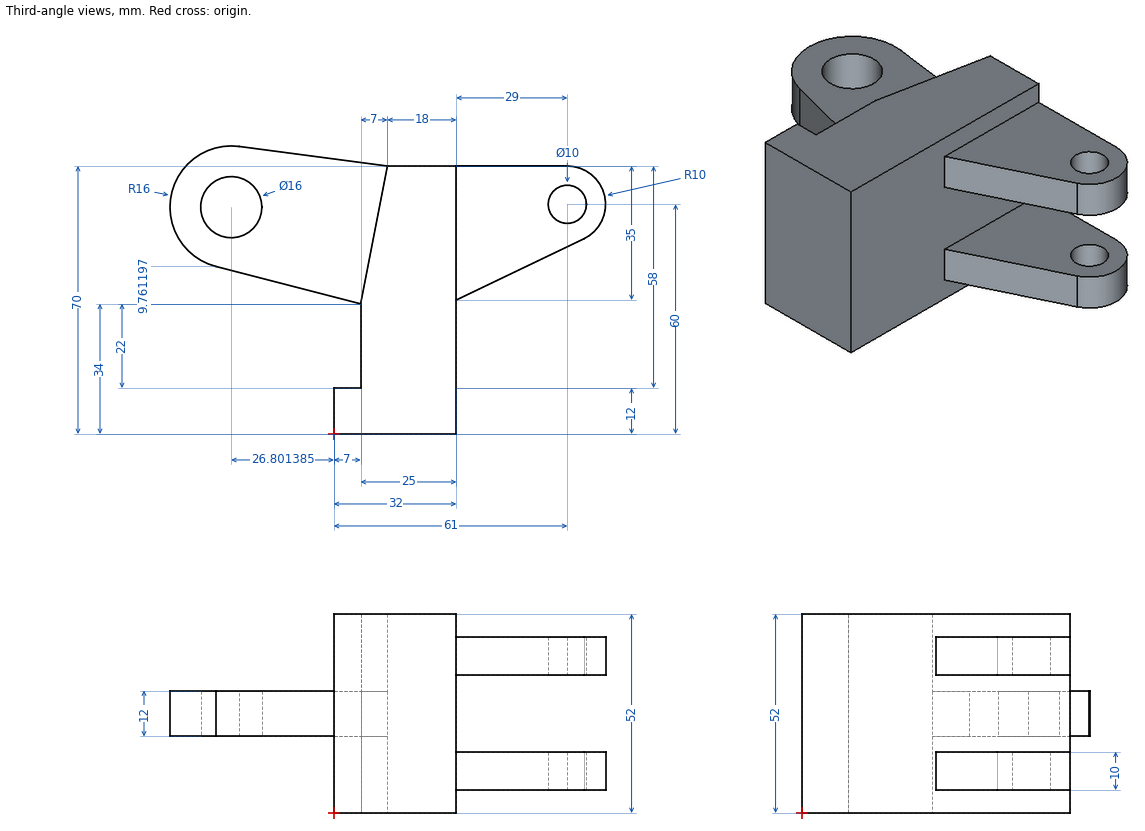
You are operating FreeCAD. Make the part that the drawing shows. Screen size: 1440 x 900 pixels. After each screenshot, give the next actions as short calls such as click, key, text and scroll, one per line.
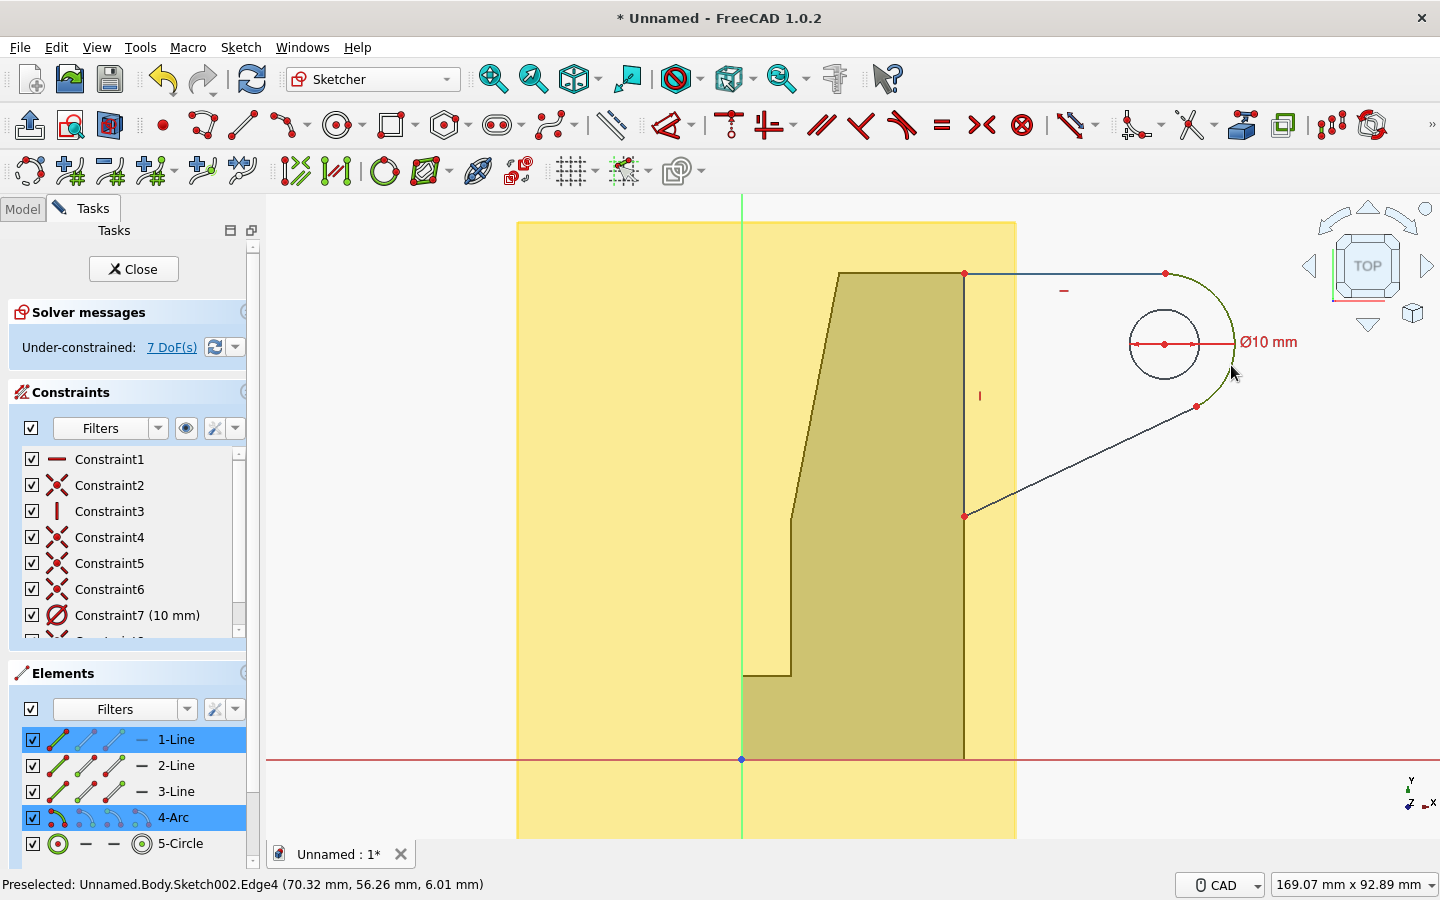
click(902, 126)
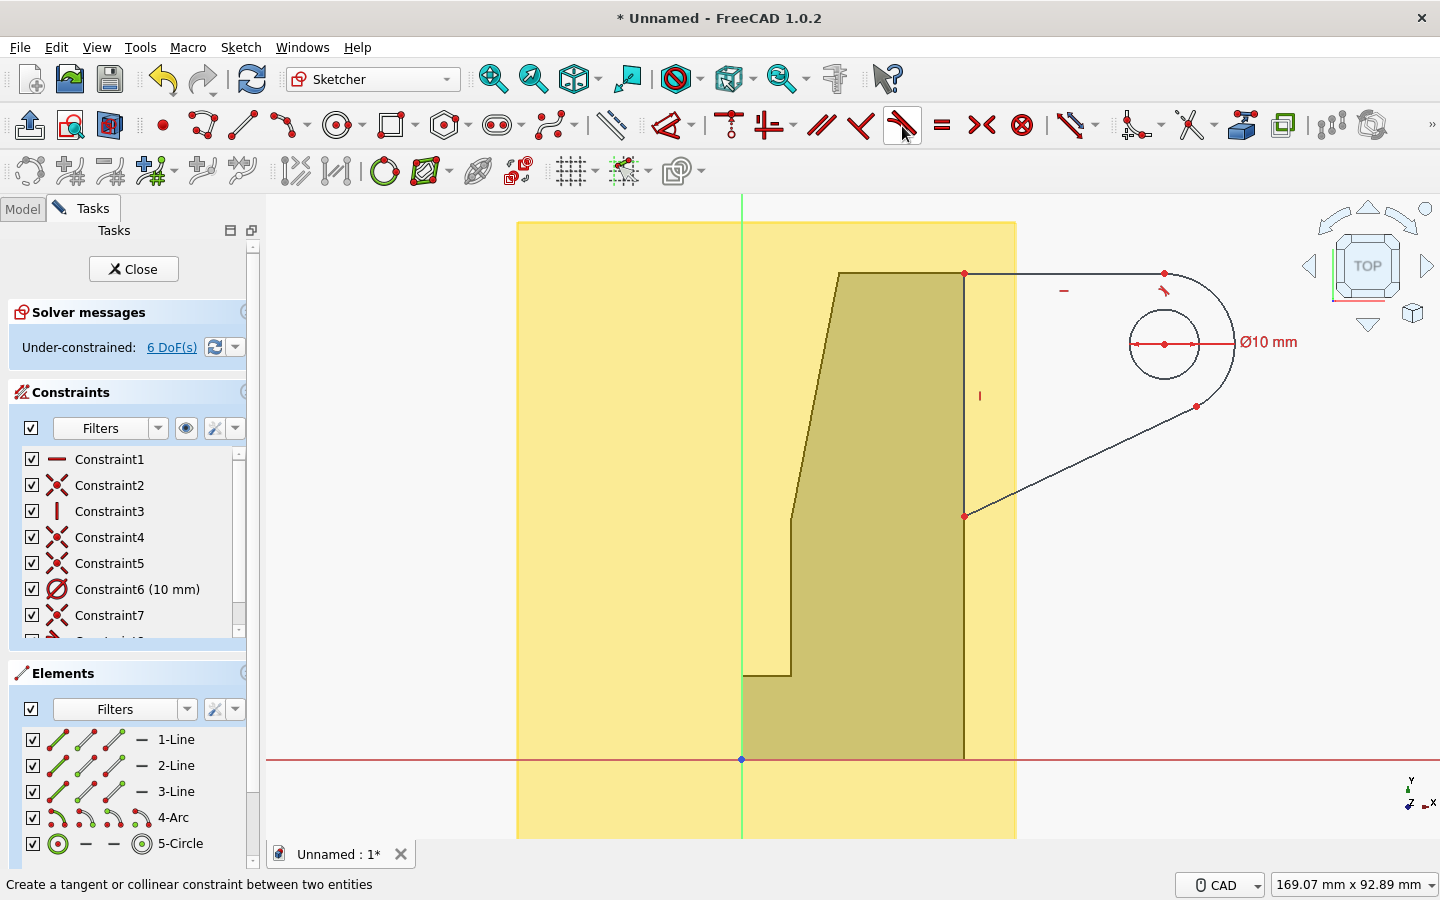
click(1034, 484)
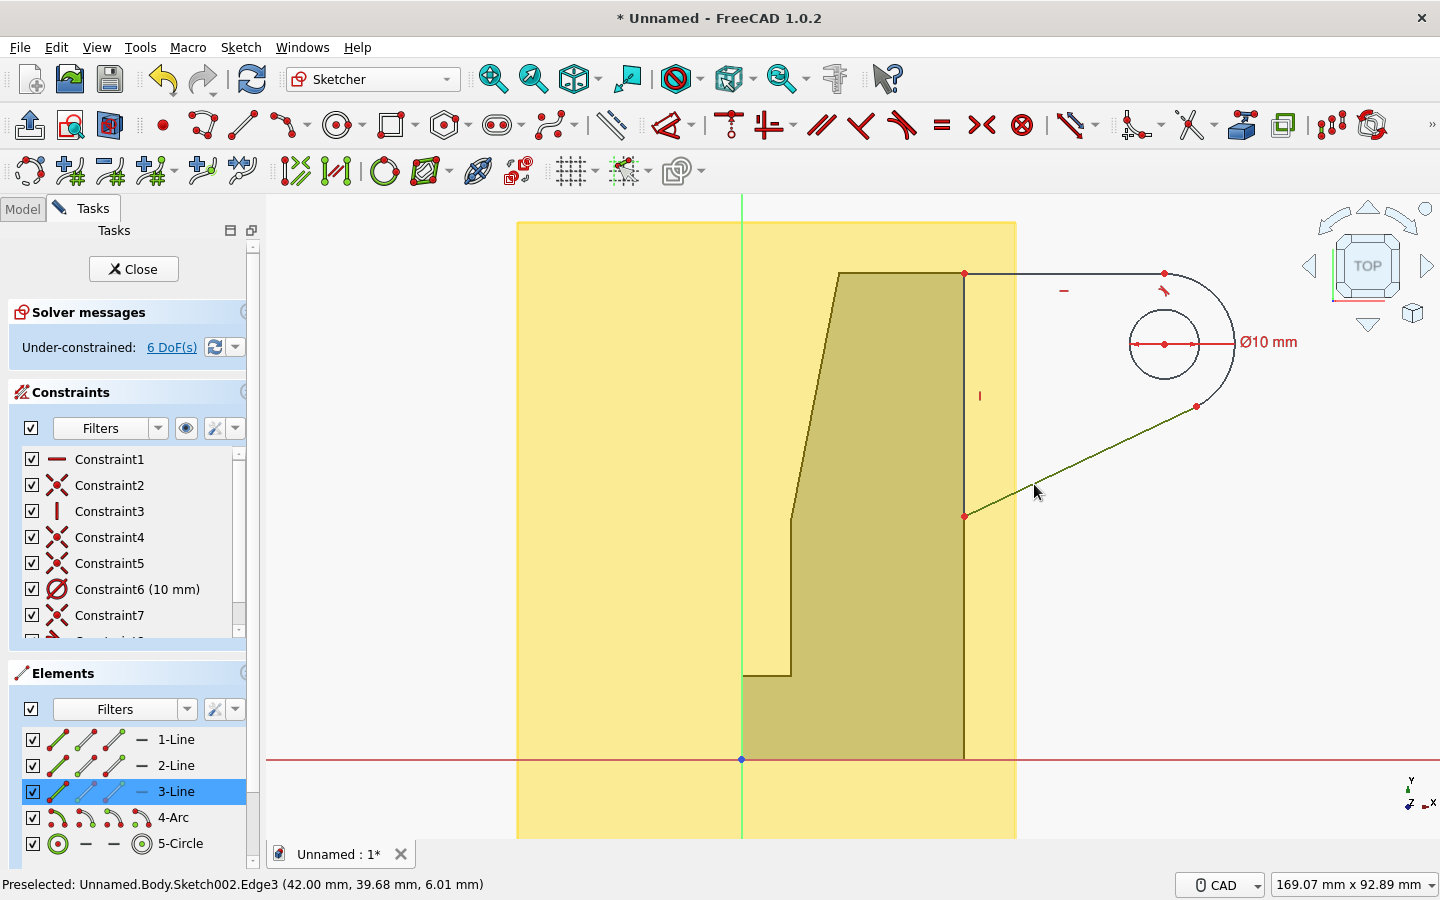
click(1231, 365)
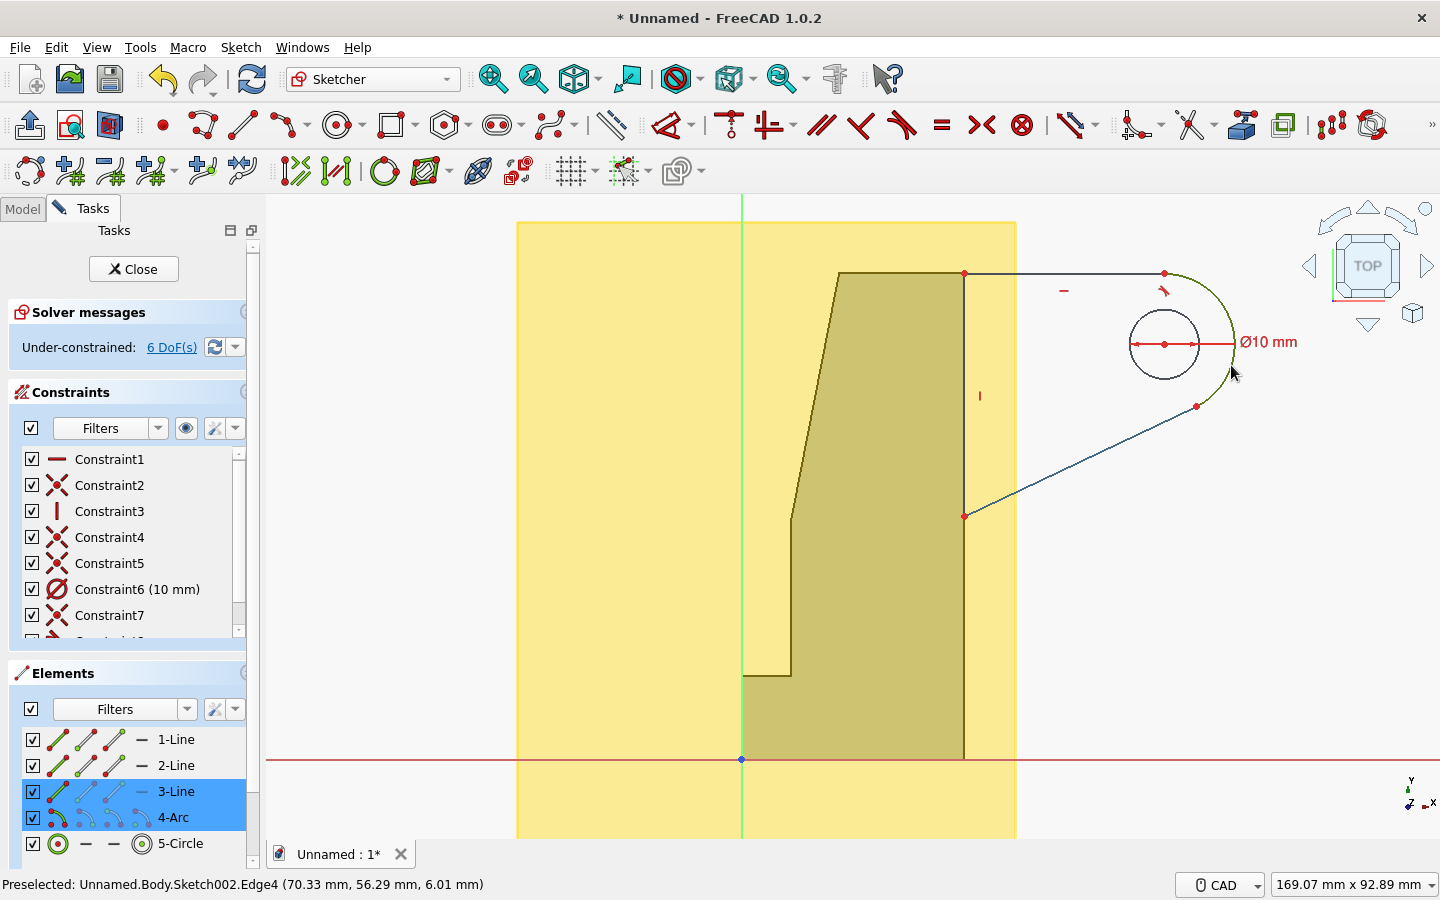
click(902, 126)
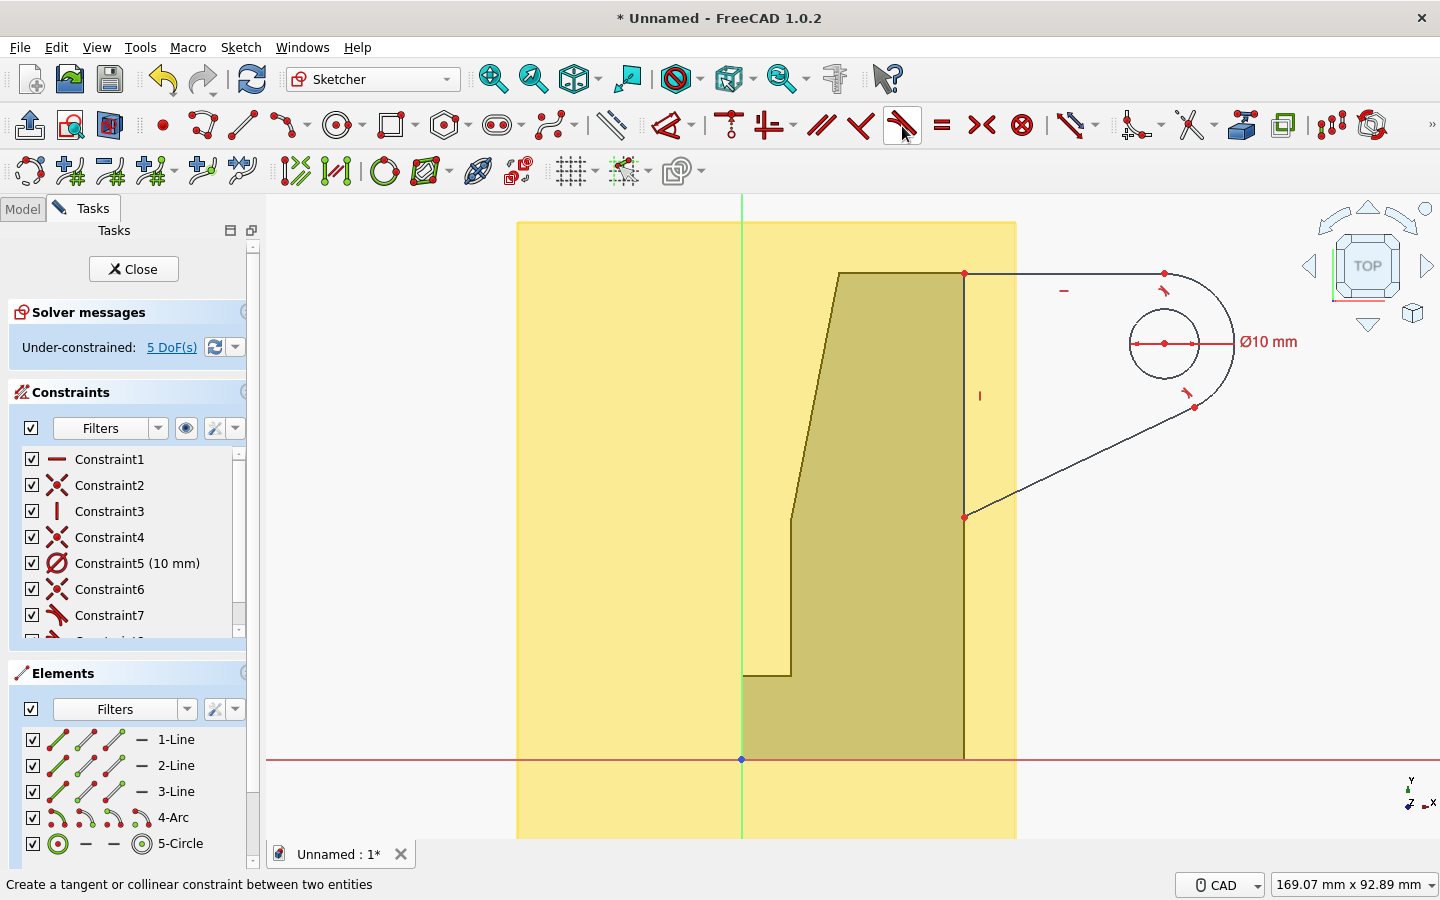
click(666, 126)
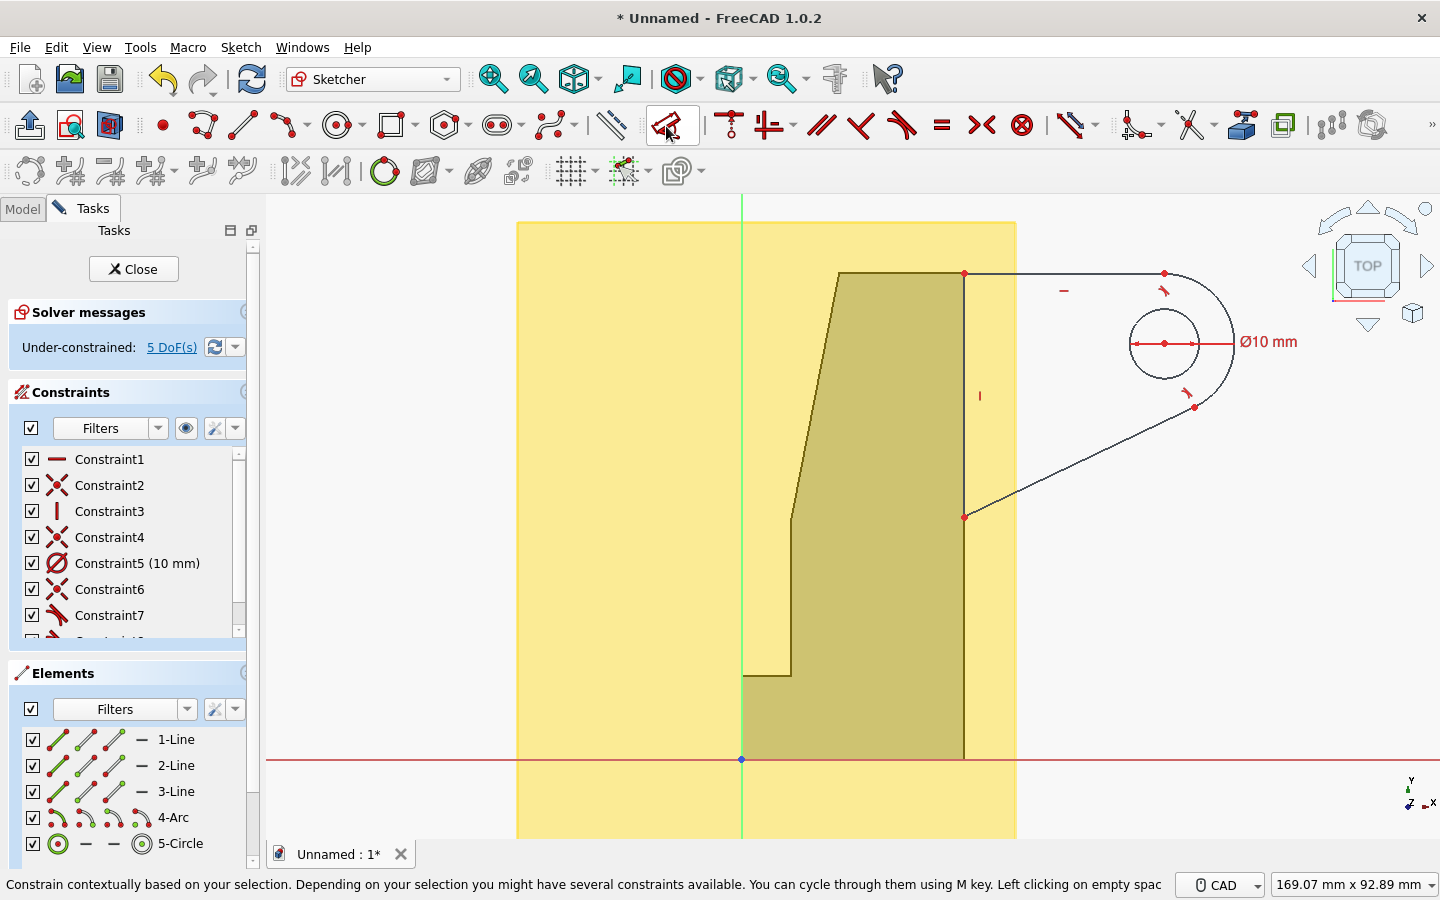
click(1231, 366)
click(1261, 376)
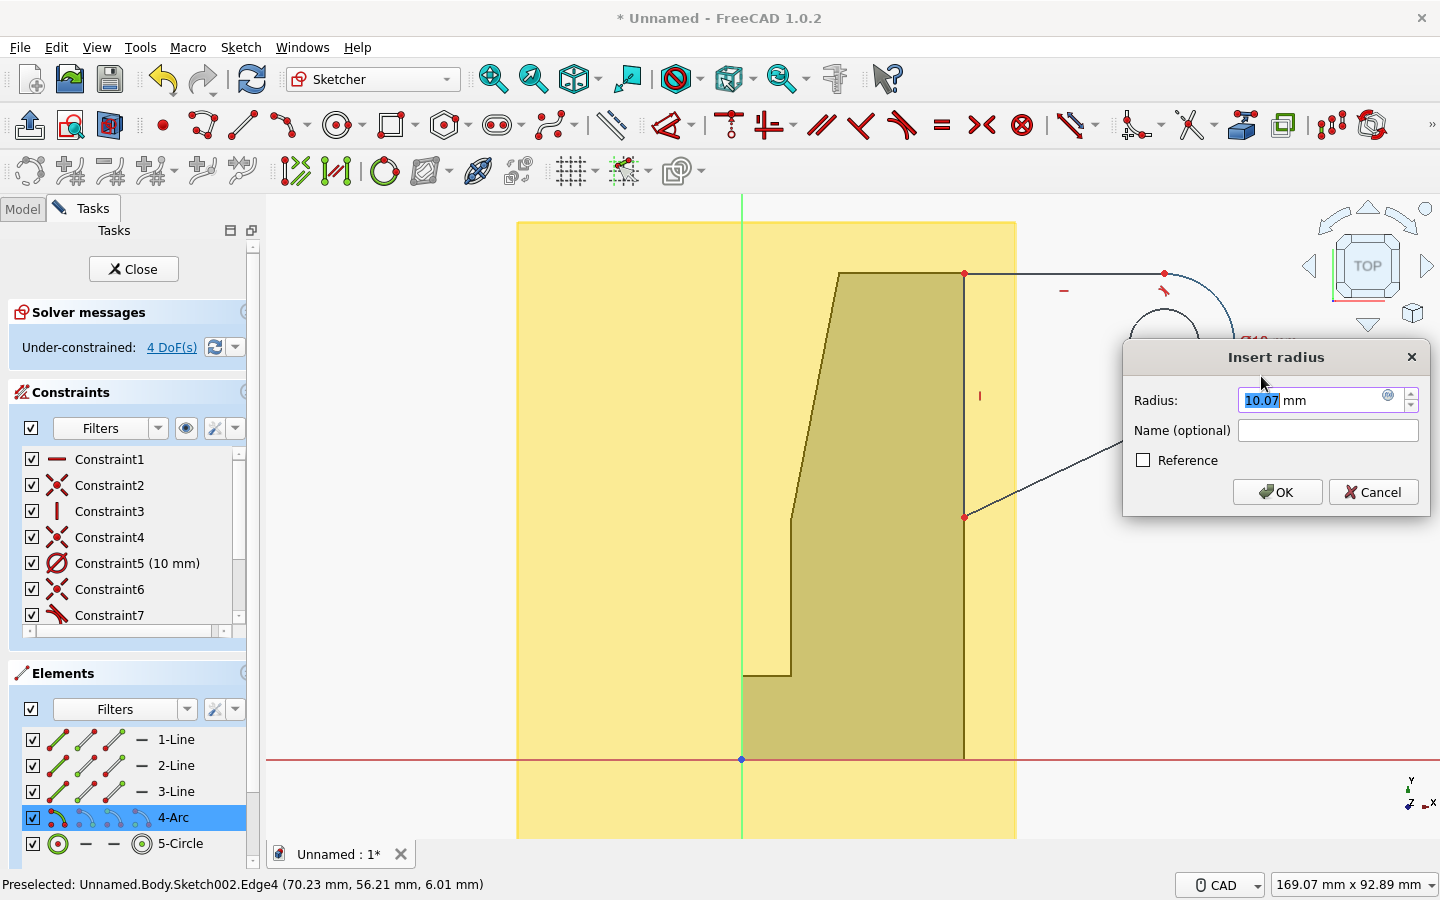
text(10)
key(Return)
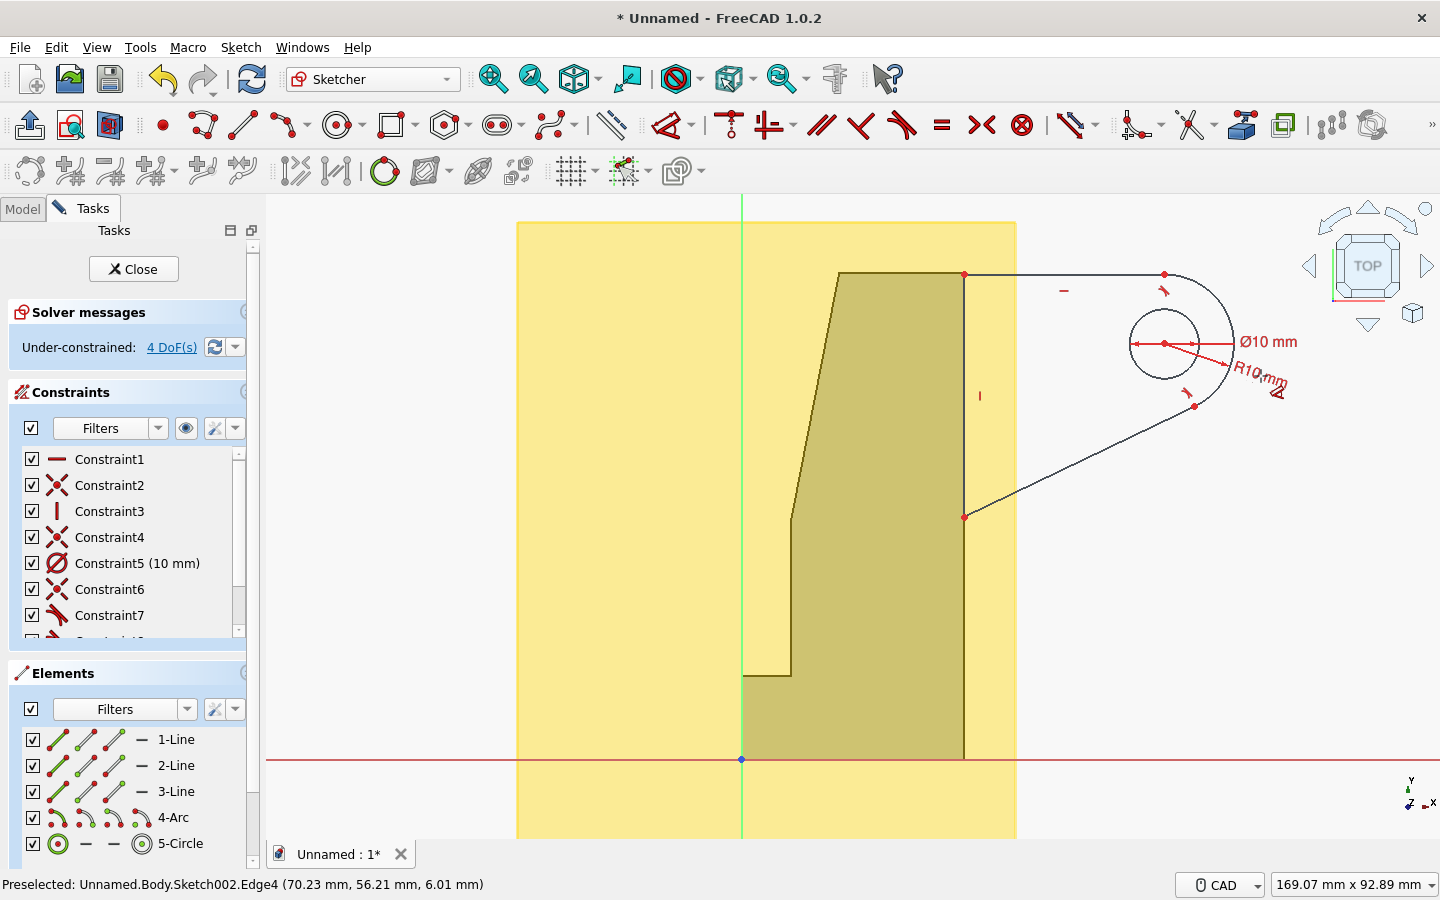
click(1104, 275)
click(1064, 241)